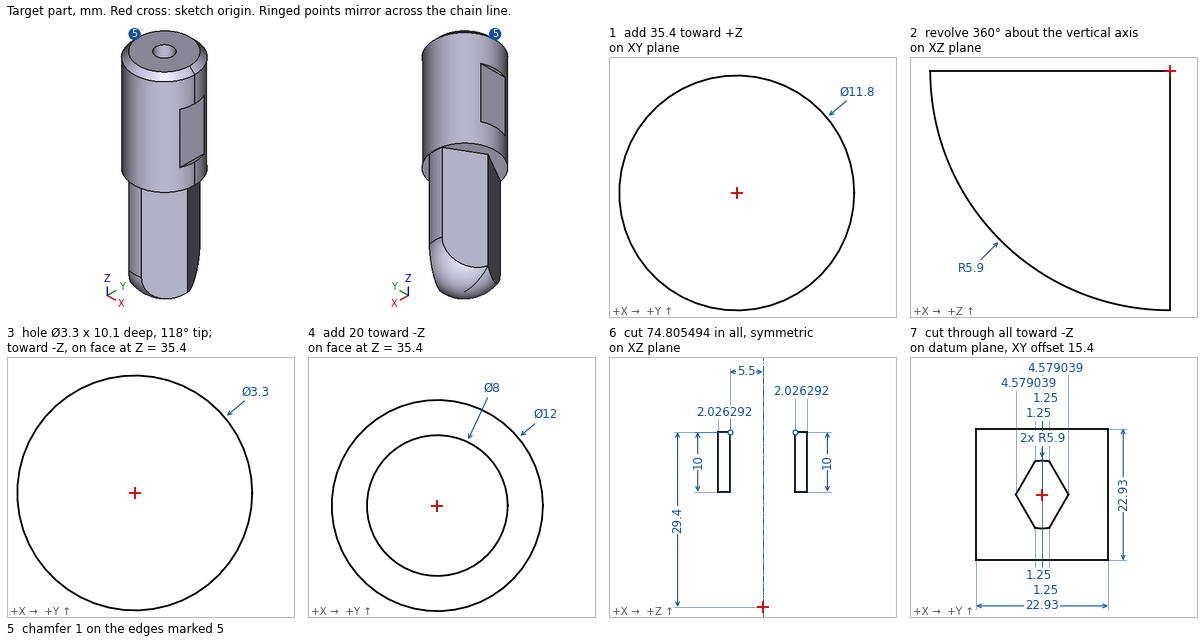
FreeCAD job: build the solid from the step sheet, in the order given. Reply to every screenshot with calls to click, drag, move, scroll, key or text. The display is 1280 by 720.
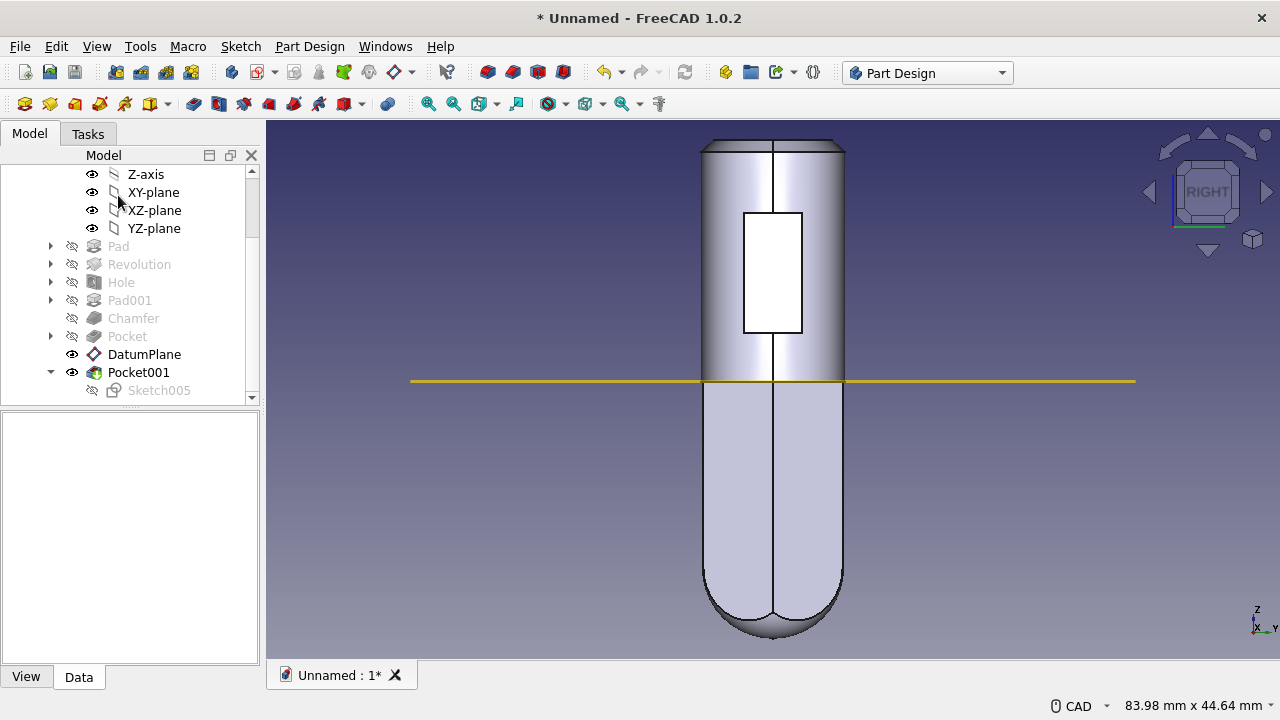
click(117, 354)
key(space)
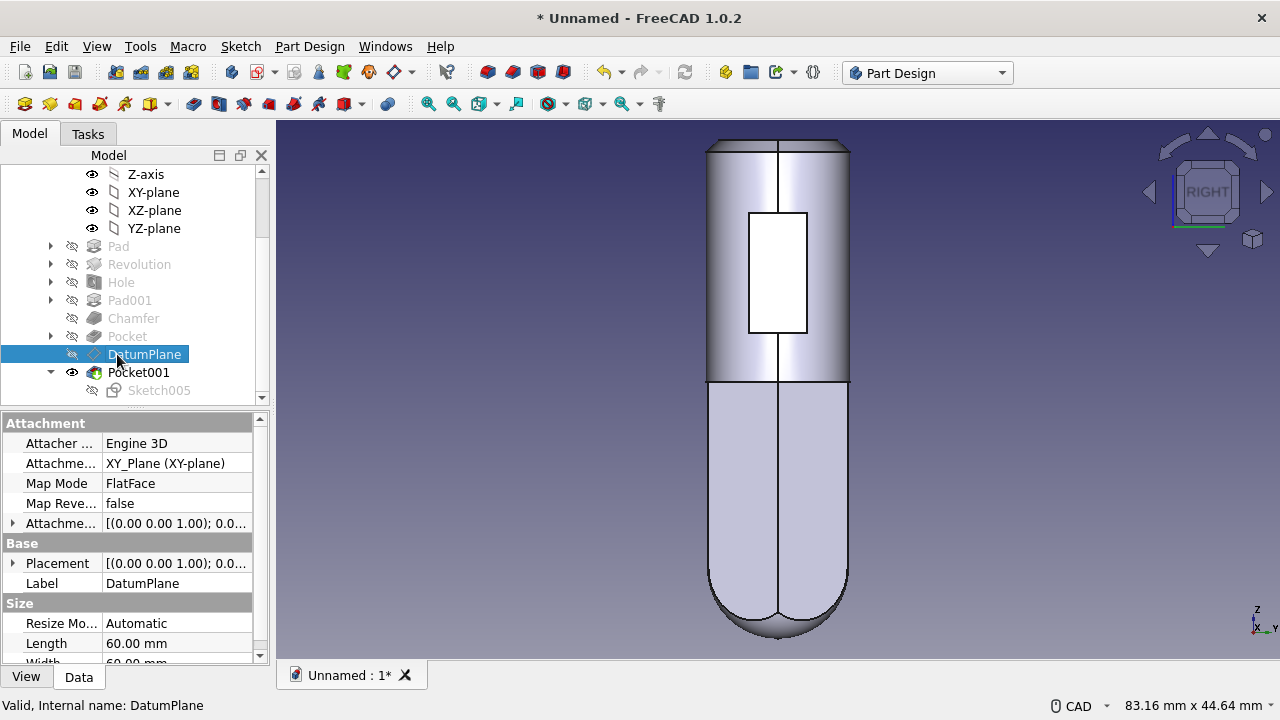
key(0)